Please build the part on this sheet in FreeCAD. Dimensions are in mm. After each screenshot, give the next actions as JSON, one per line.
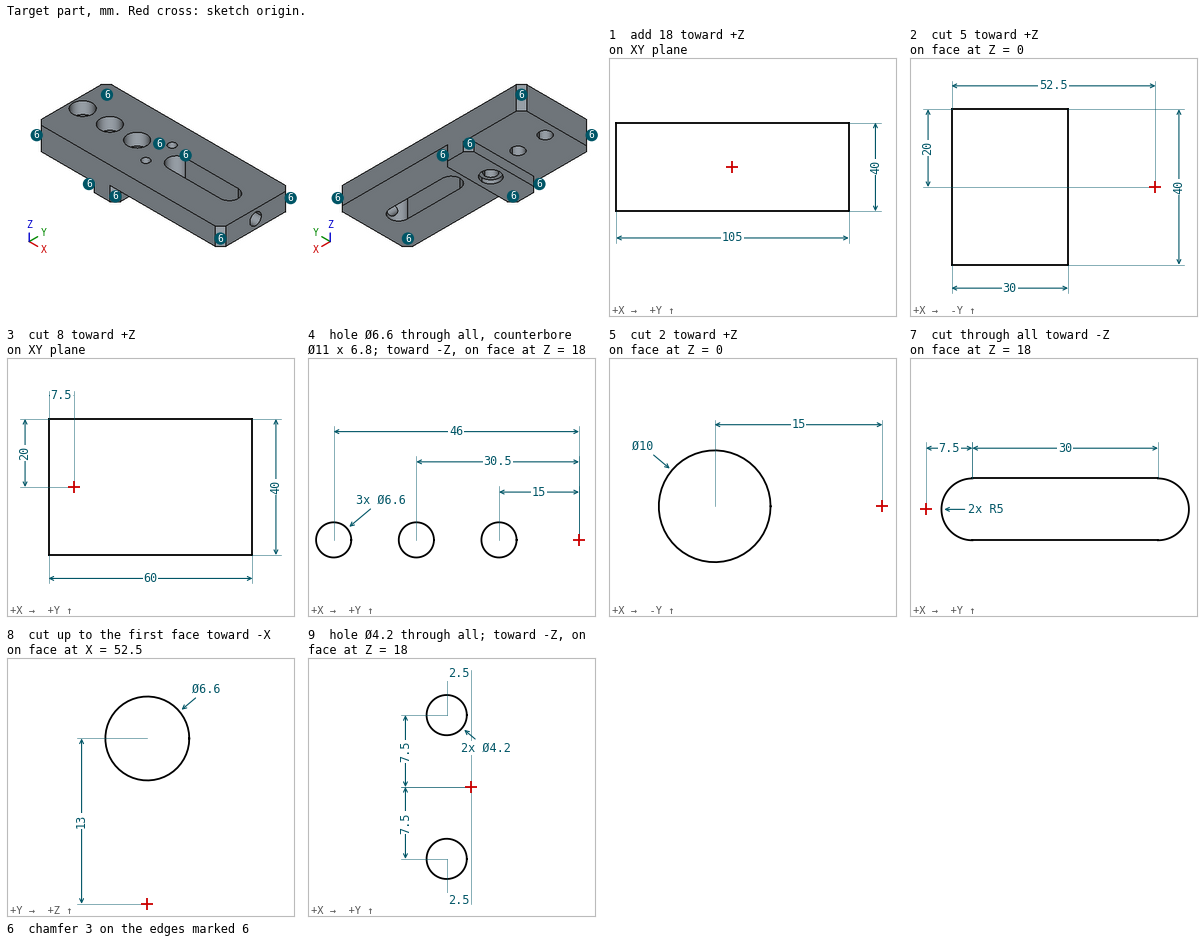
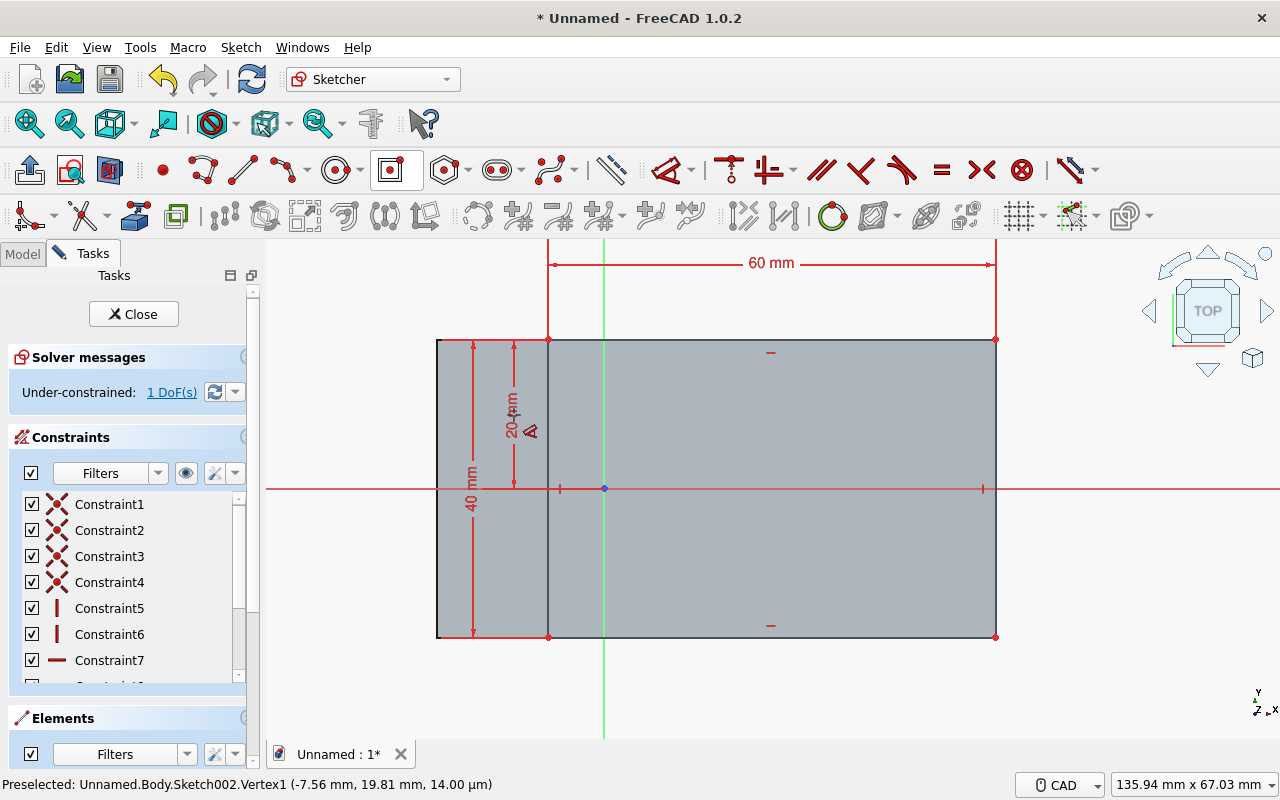
{"action": "left_click", "coordinate": [548, 340]}
{"action": "left_click", "coordinate": [576, 306]}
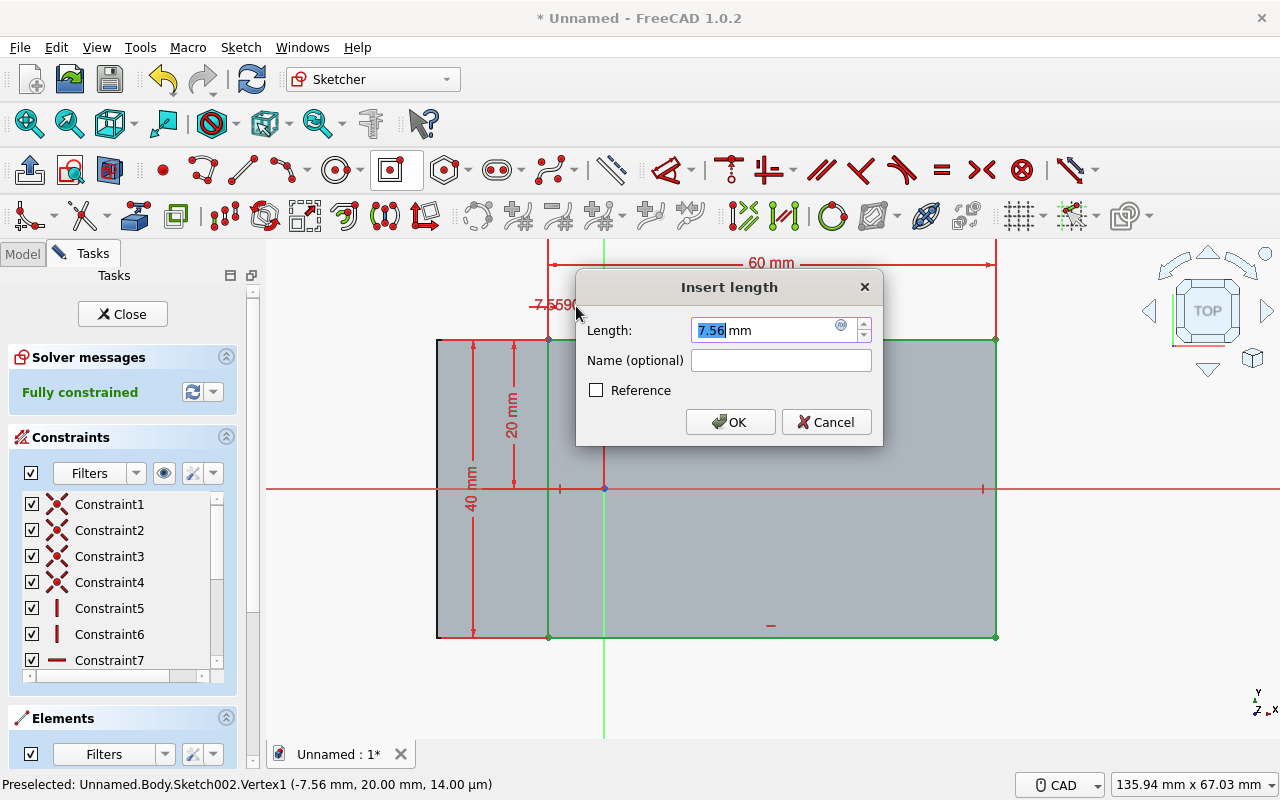
{"action": "type", "text": "7.5"}
{"action": "key", "text": "Return"}
{"action": "key", "text": "Escape"}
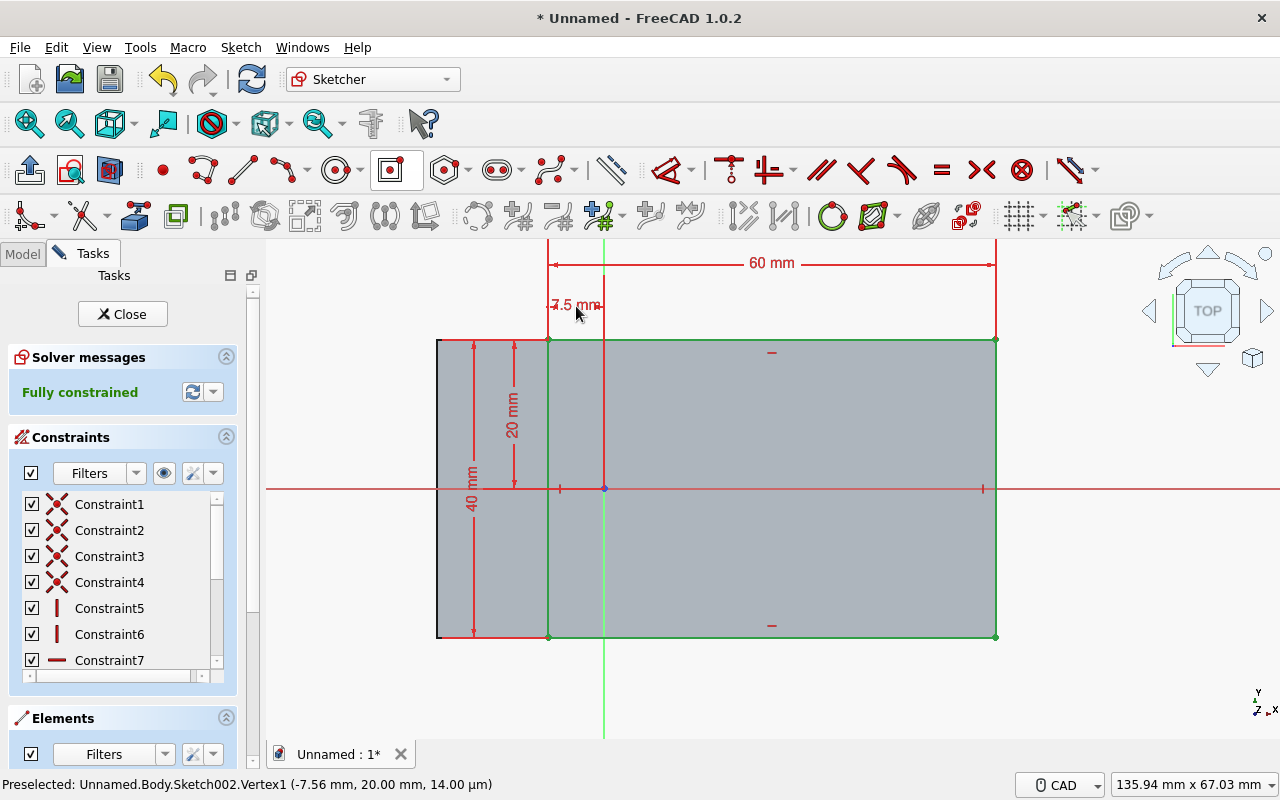
{"action": "left_click", "coordinate": [123, 314]}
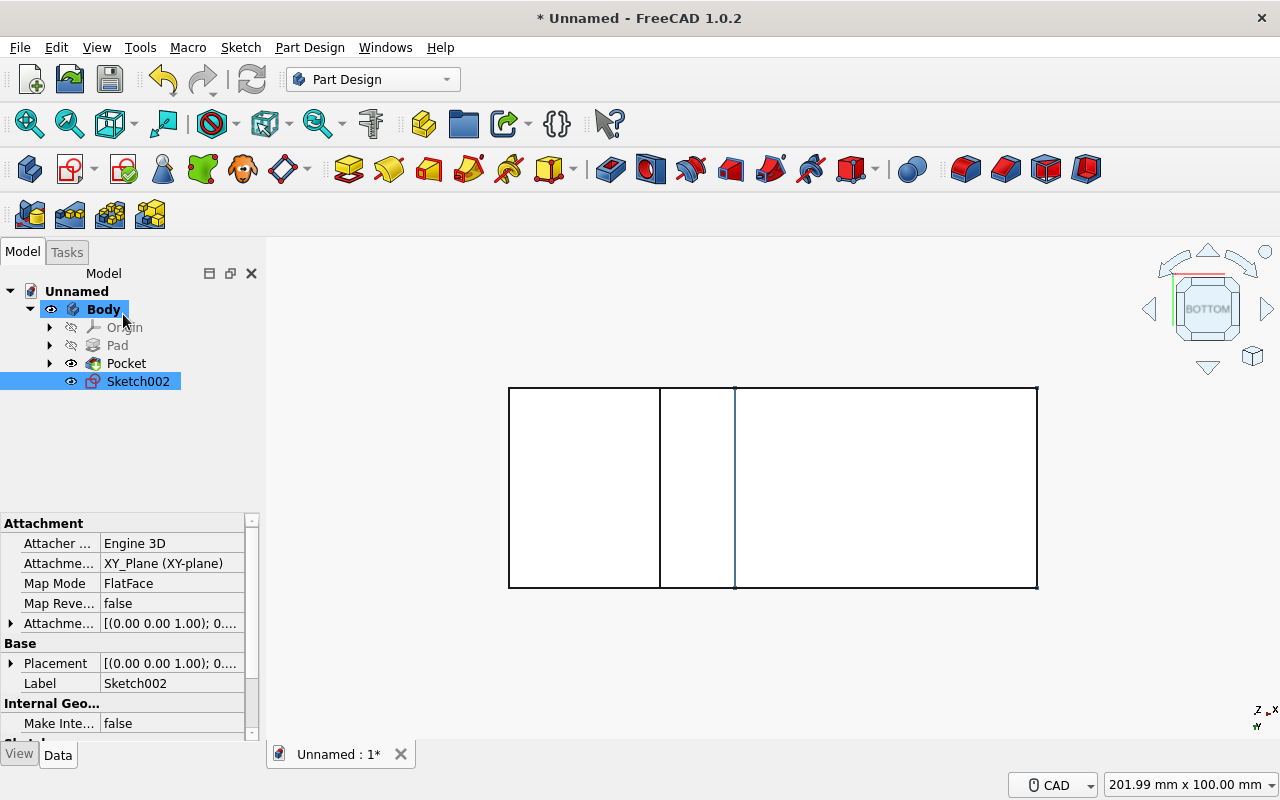
{"action": "left_click", "coordinate": [612, 170]}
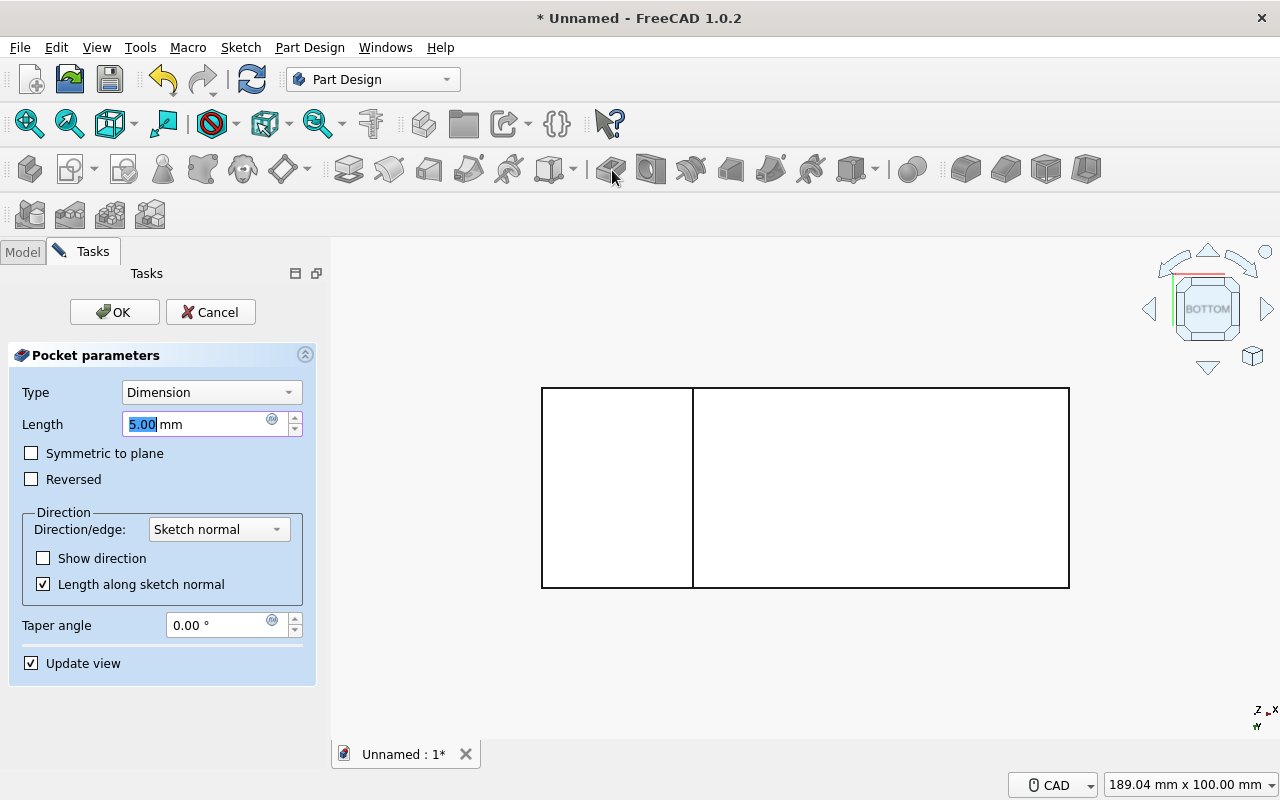
{"action": "type", "text": "8"}
{"action": "key", "text": "Tab"}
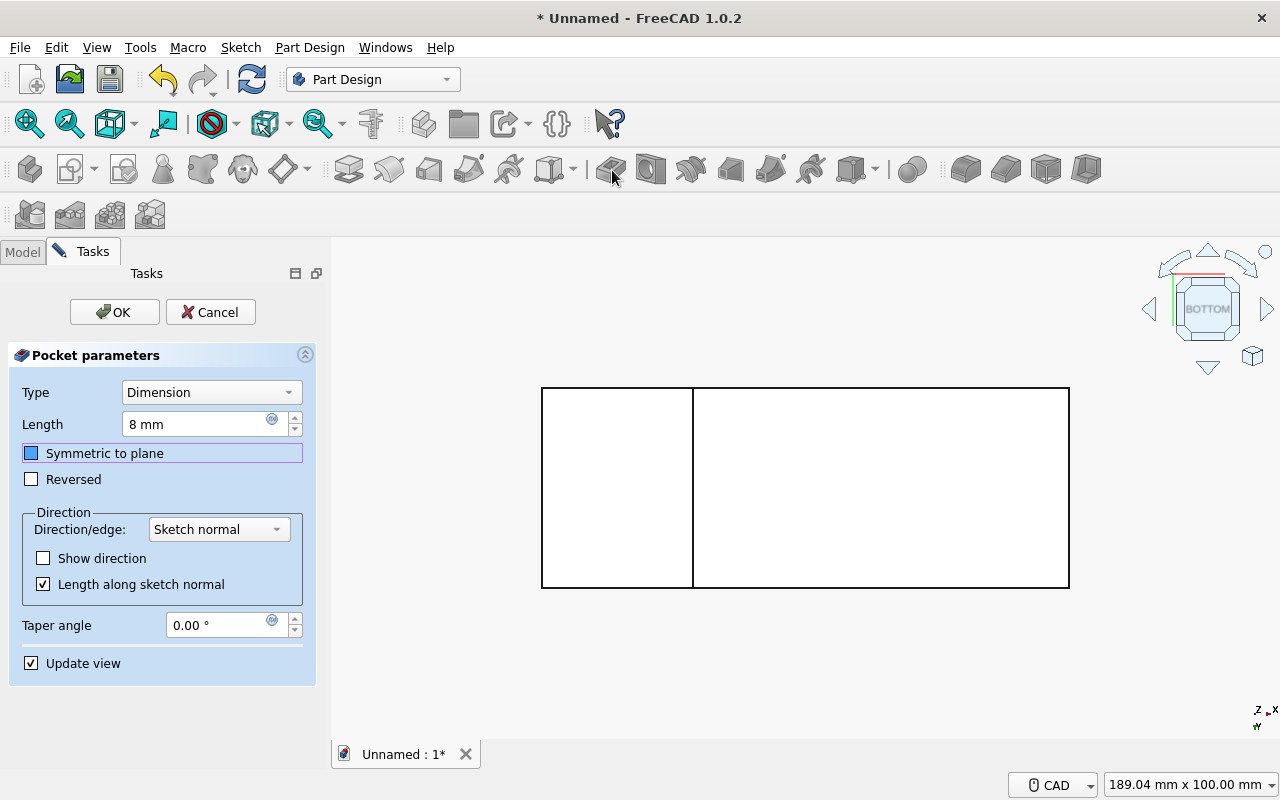
{"action": "left_click", "coordinate": [30, 479]}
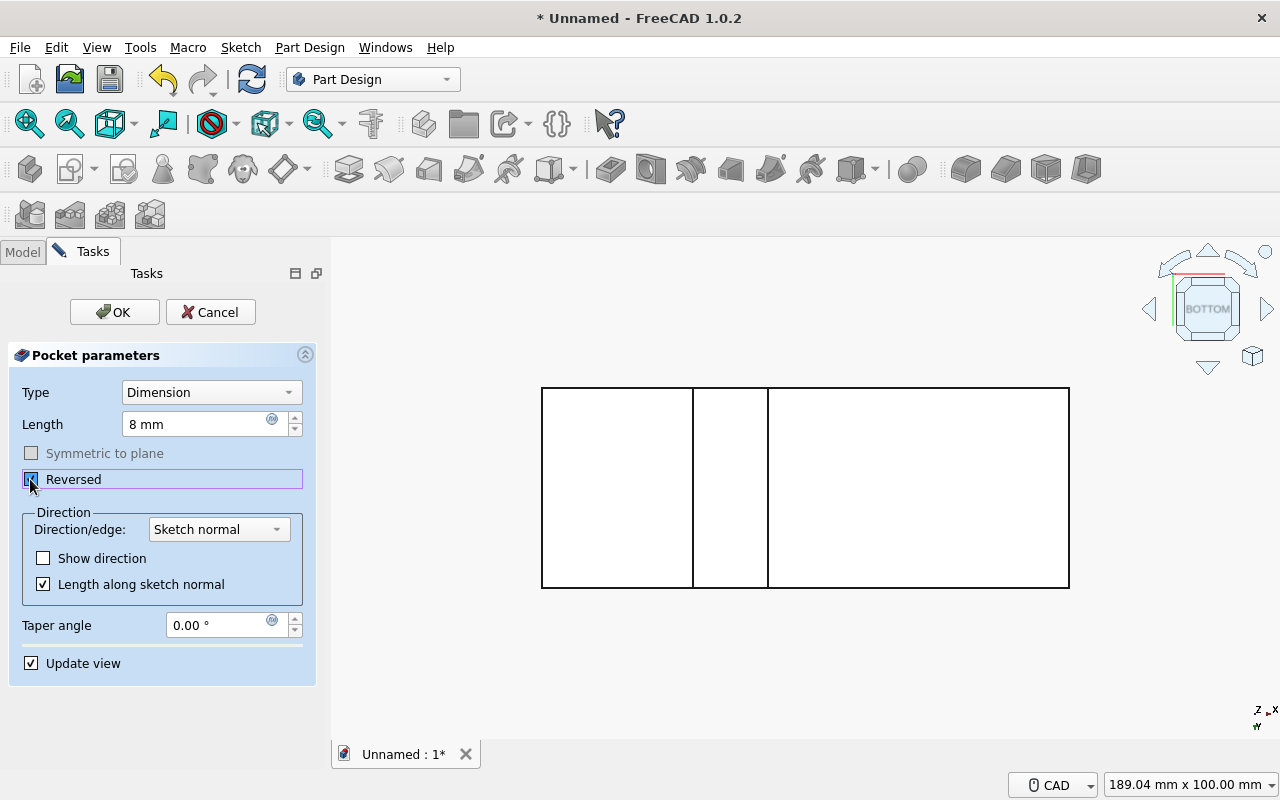
{"action": "left_click", "coordinate": [115, 312]}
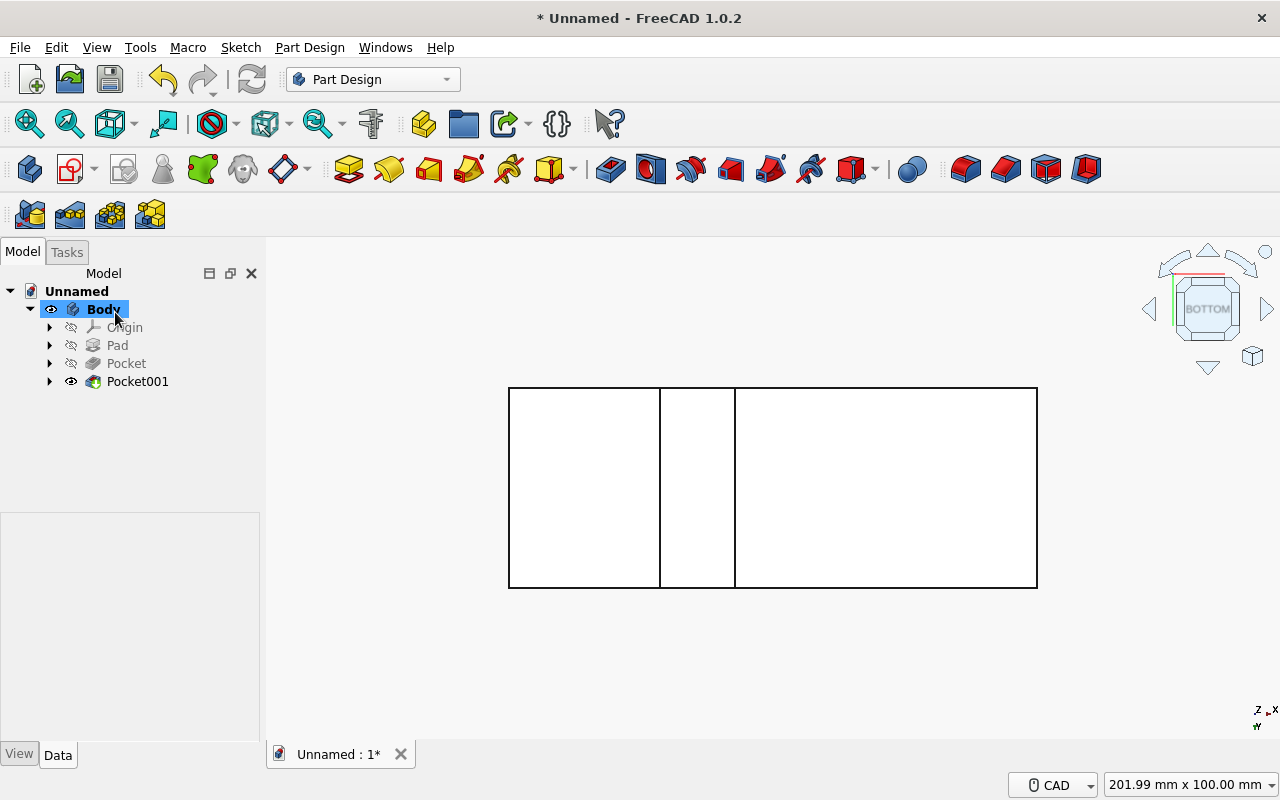
{"action": "key", "text": "0"}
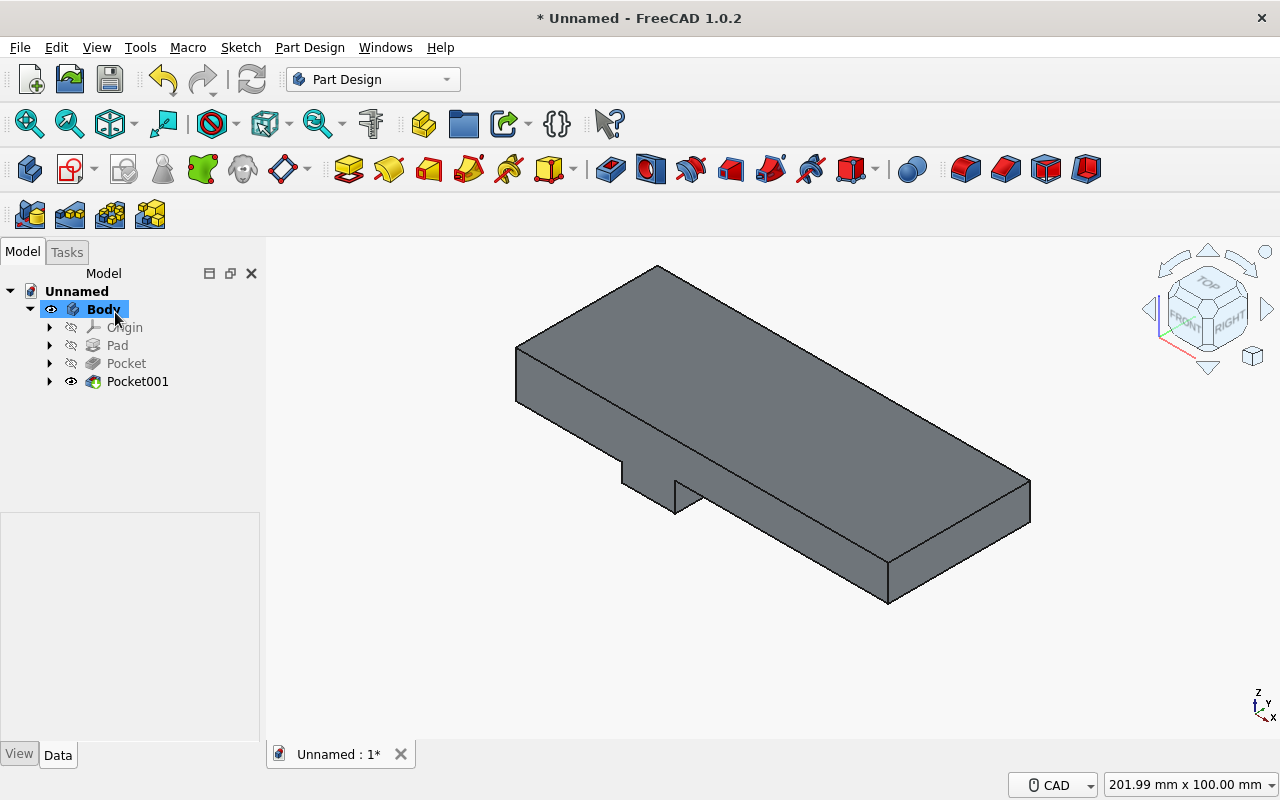
{"action": "left_click", "coordinate": [879, 475]}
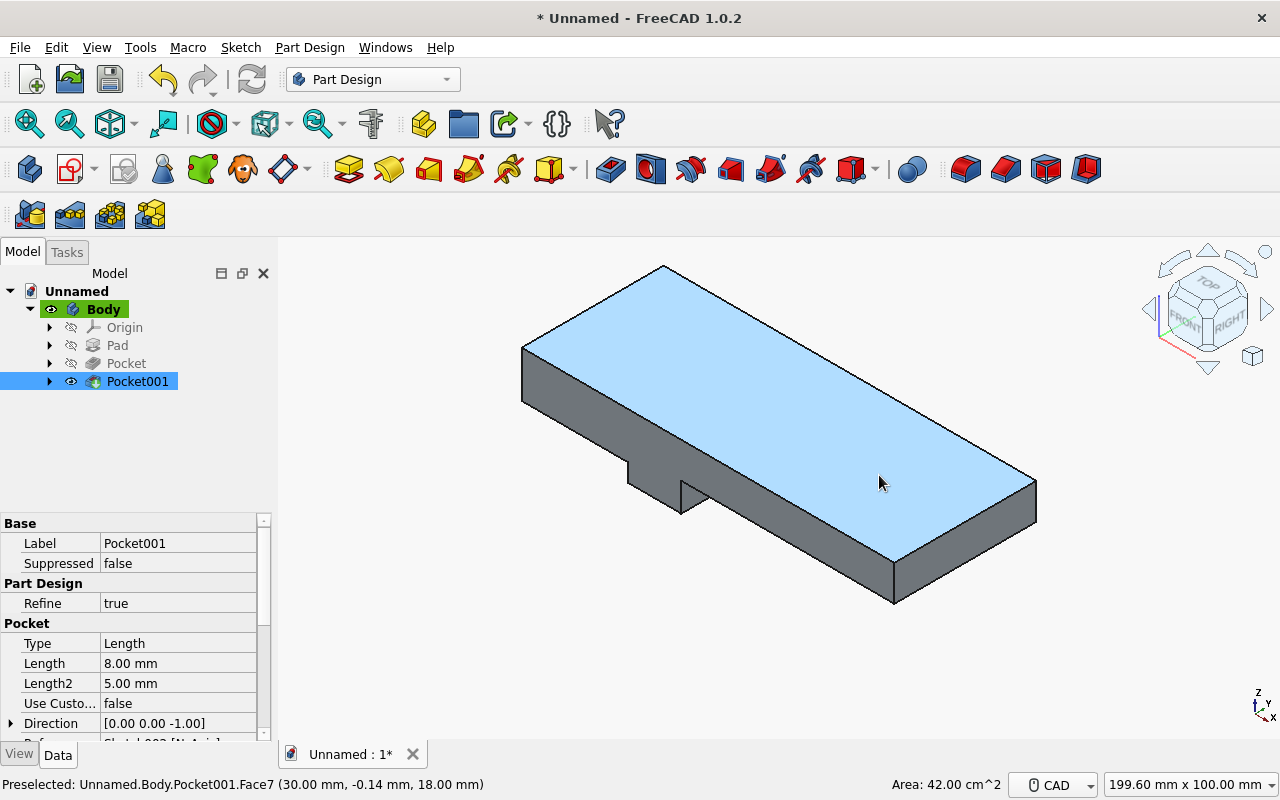
{"action": "left_click", "coordinate": [70, 170]}